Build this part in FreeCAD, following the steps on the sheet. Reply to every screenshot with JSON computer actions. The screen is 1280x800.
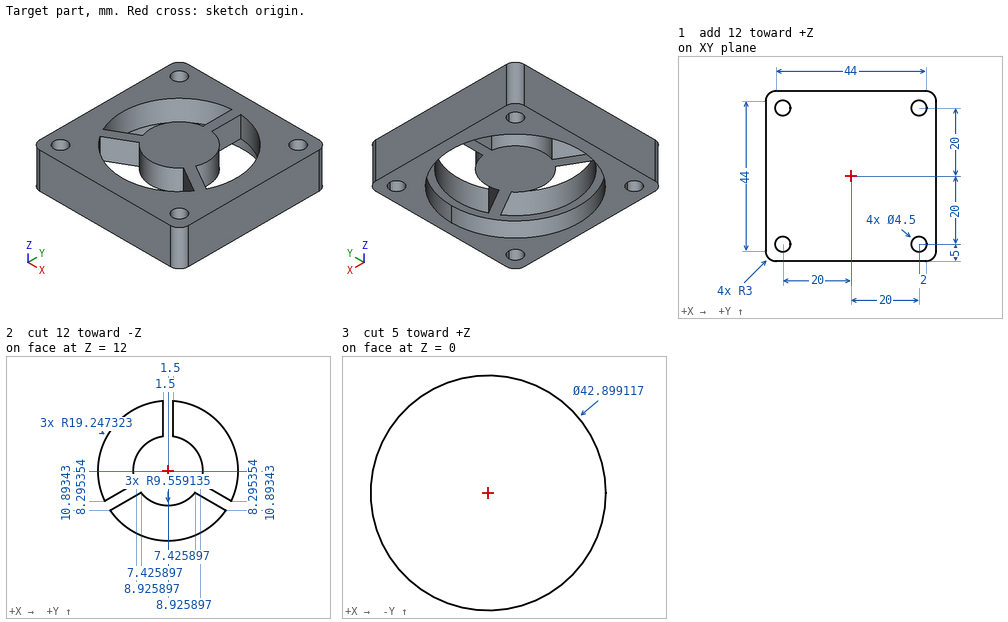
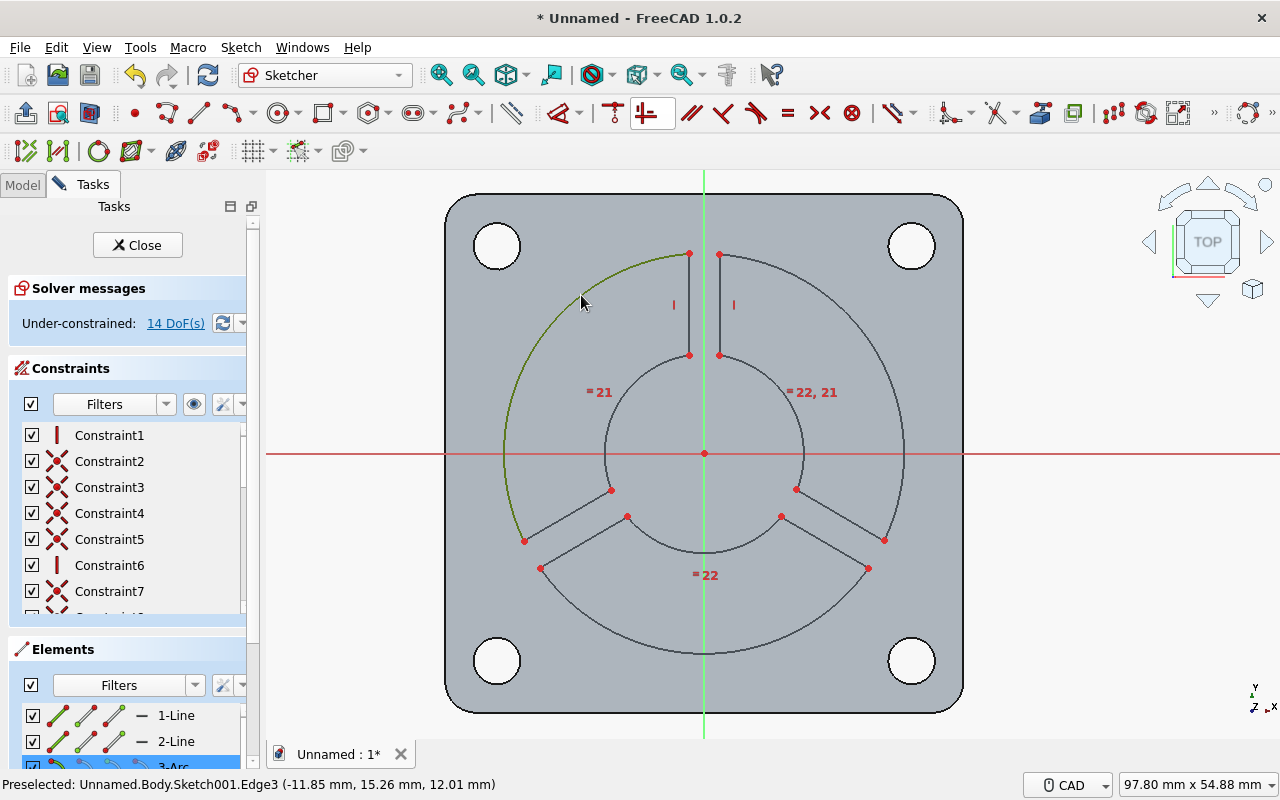
{"action": "left_click", "coordinate": [902, 428]}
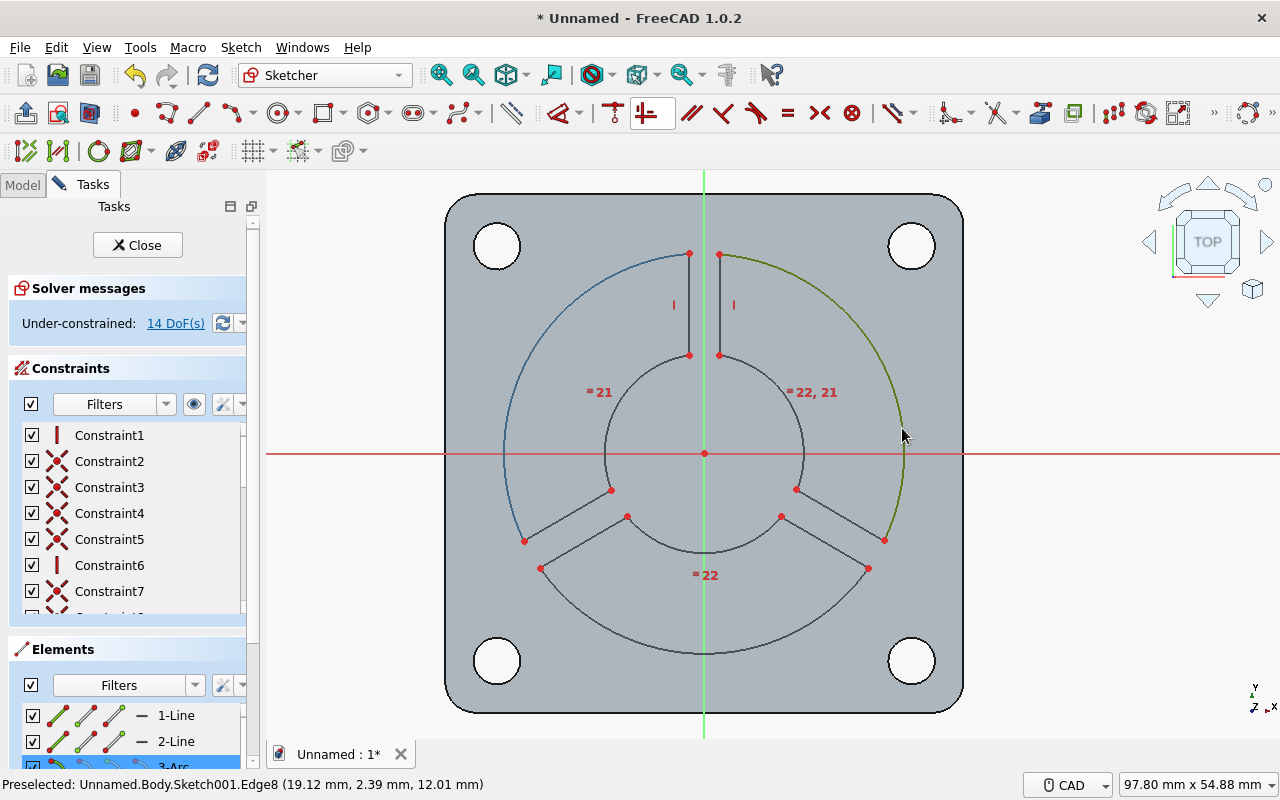
{"action": "left_click", "coordinate": [629, 639]}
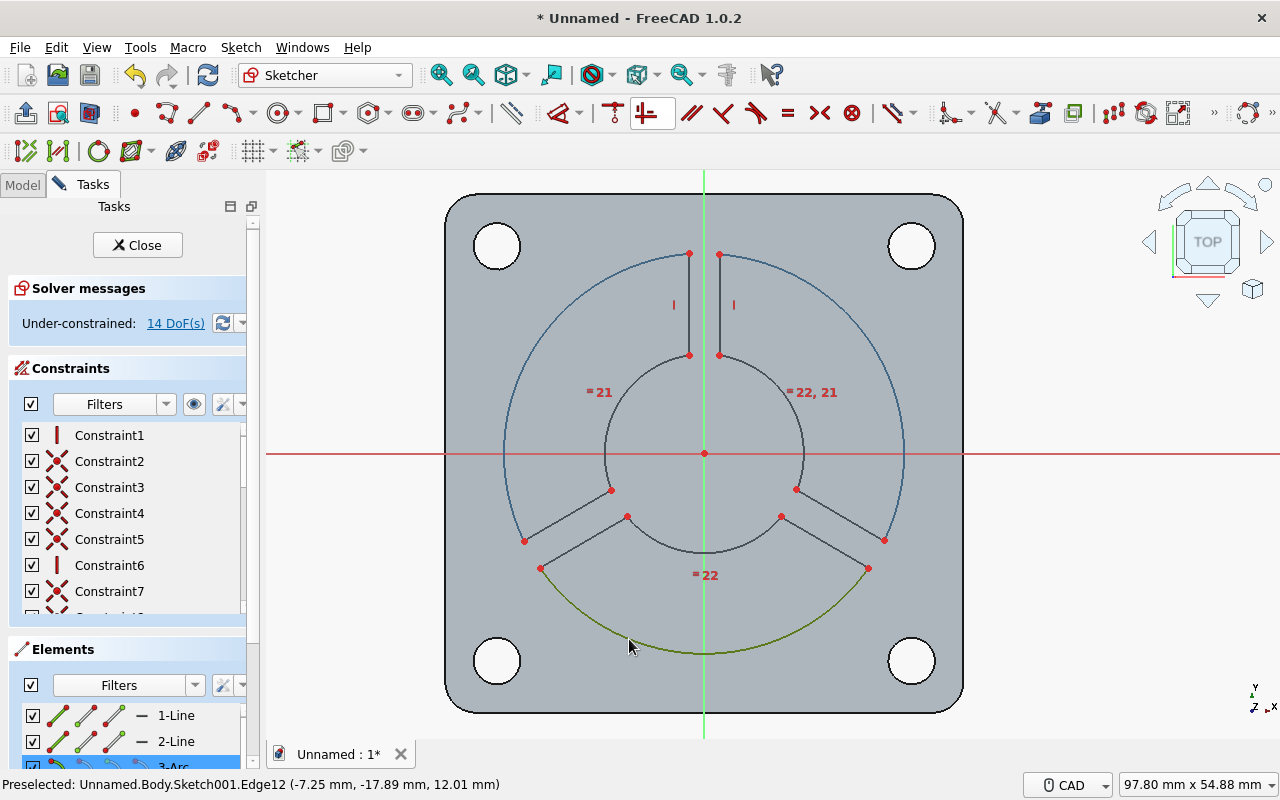
{"action": "left_click", "coordinate": [788, 114]}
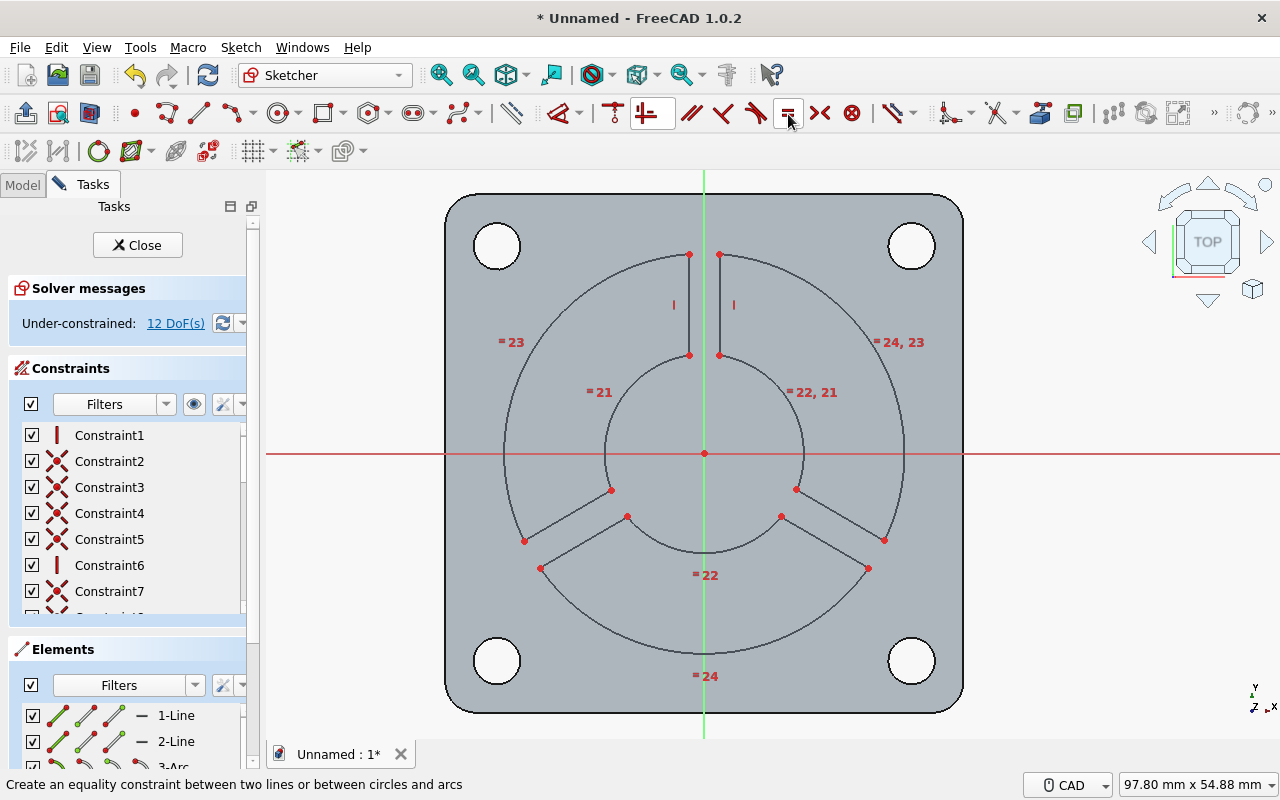
{"action": "left_click", "coordinate": [558, 114]}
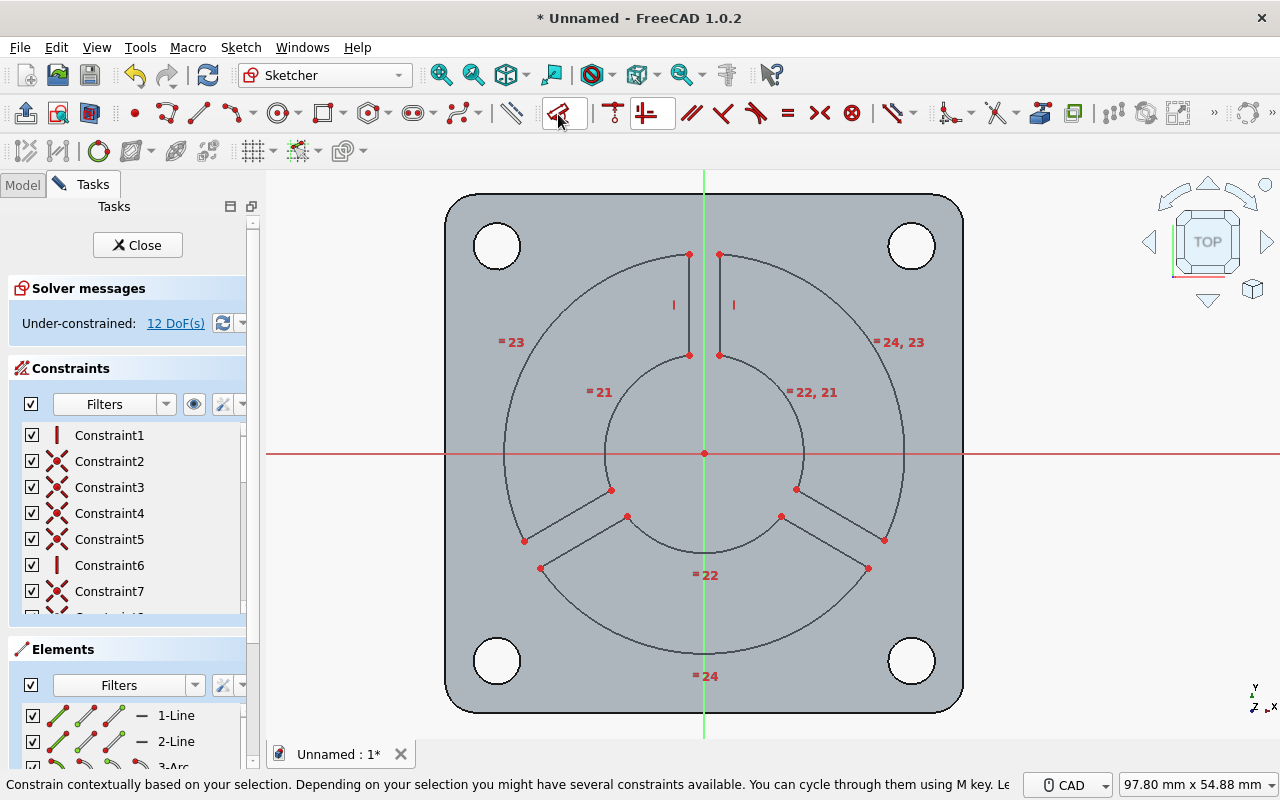
{"action": "left_click", "coordinate": [582, 296]}
{"action": "left_click", "coordinate": [562, 271]}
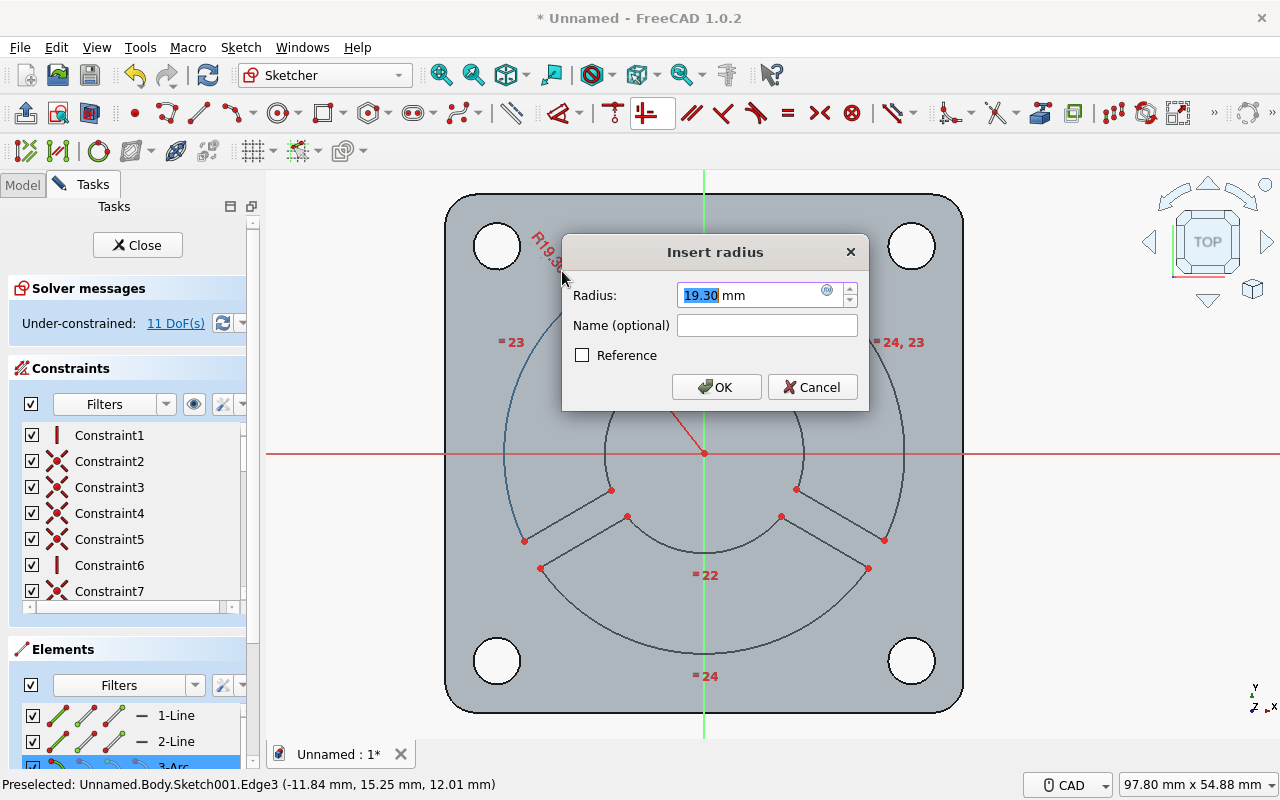
{"action": "type", "text": "19.247323"}
{"action": "key", "text": "Return"}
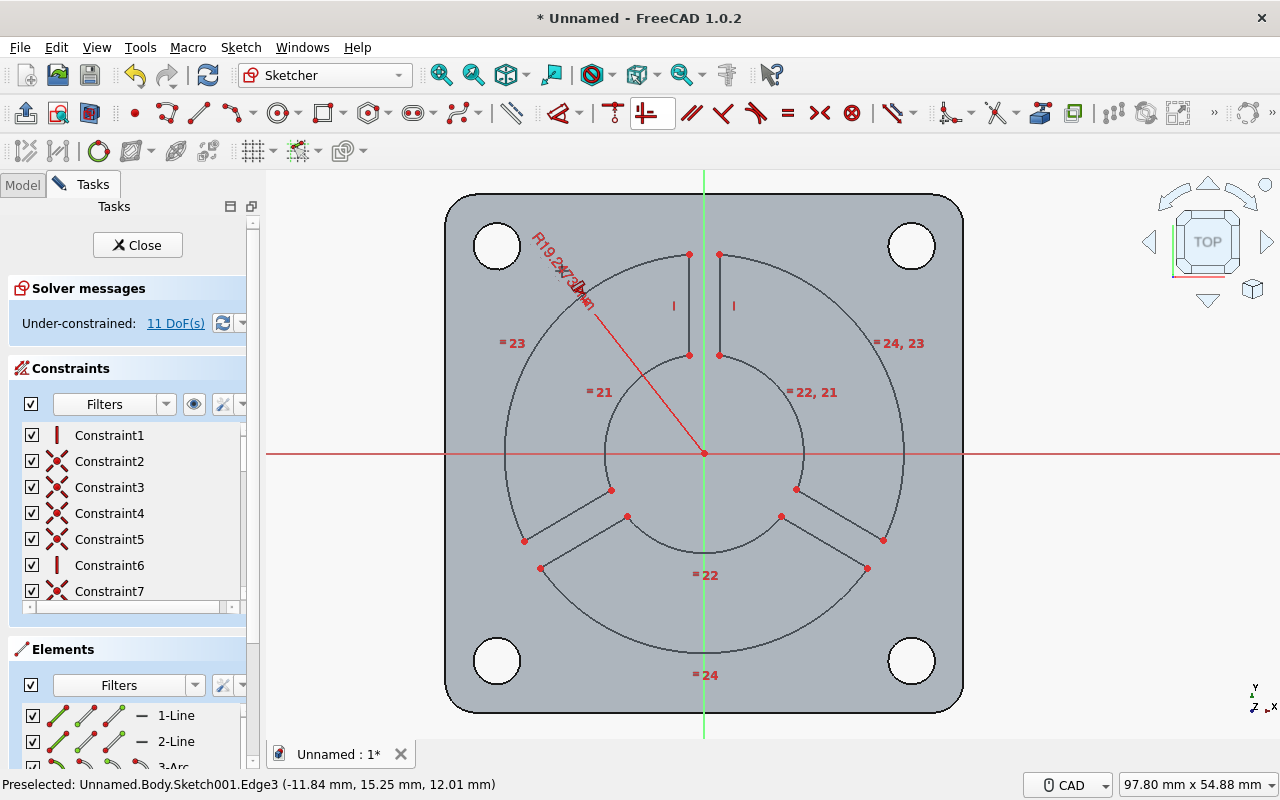
{"action": "left_click", "coordinate": [641, 377]}
{"action": "left_click", "coordinate": [621, 352]}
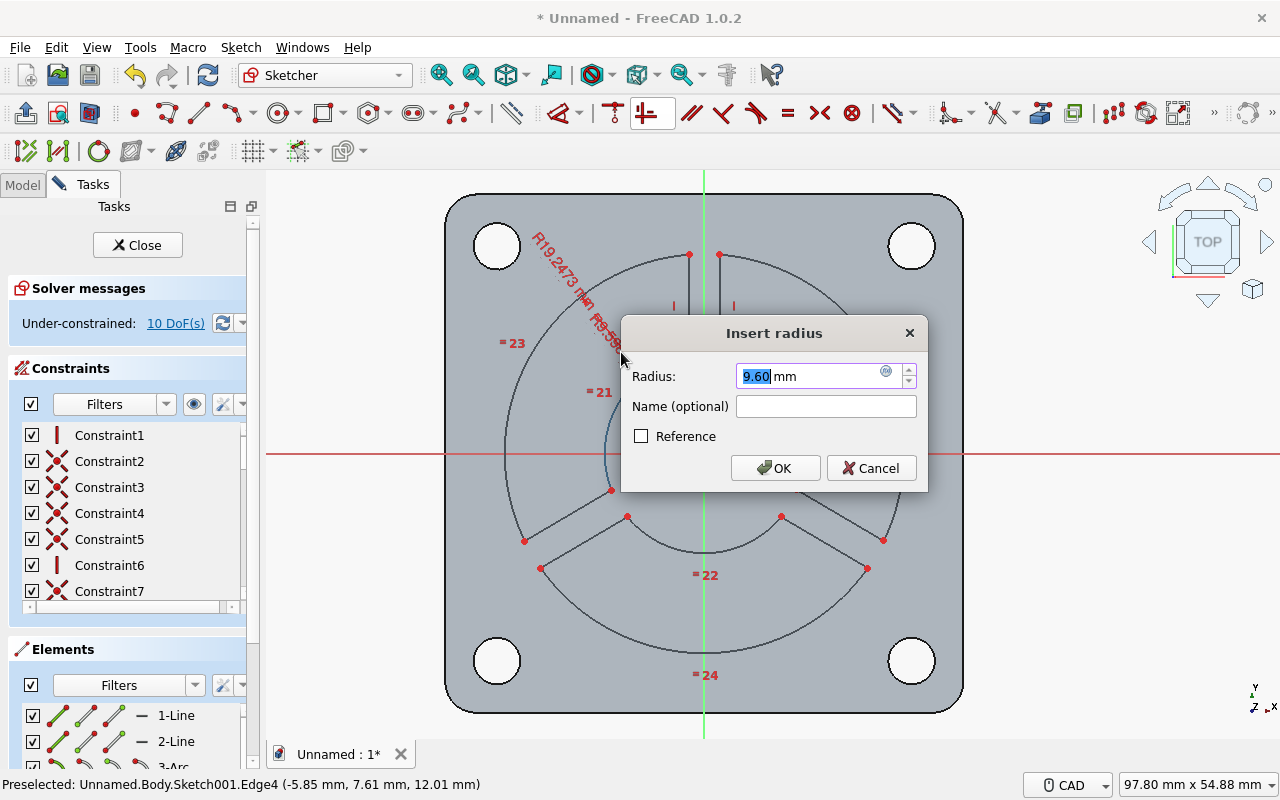
{"action": "type", "text": "9.559135"}
{"action": "key", "text": "Return"}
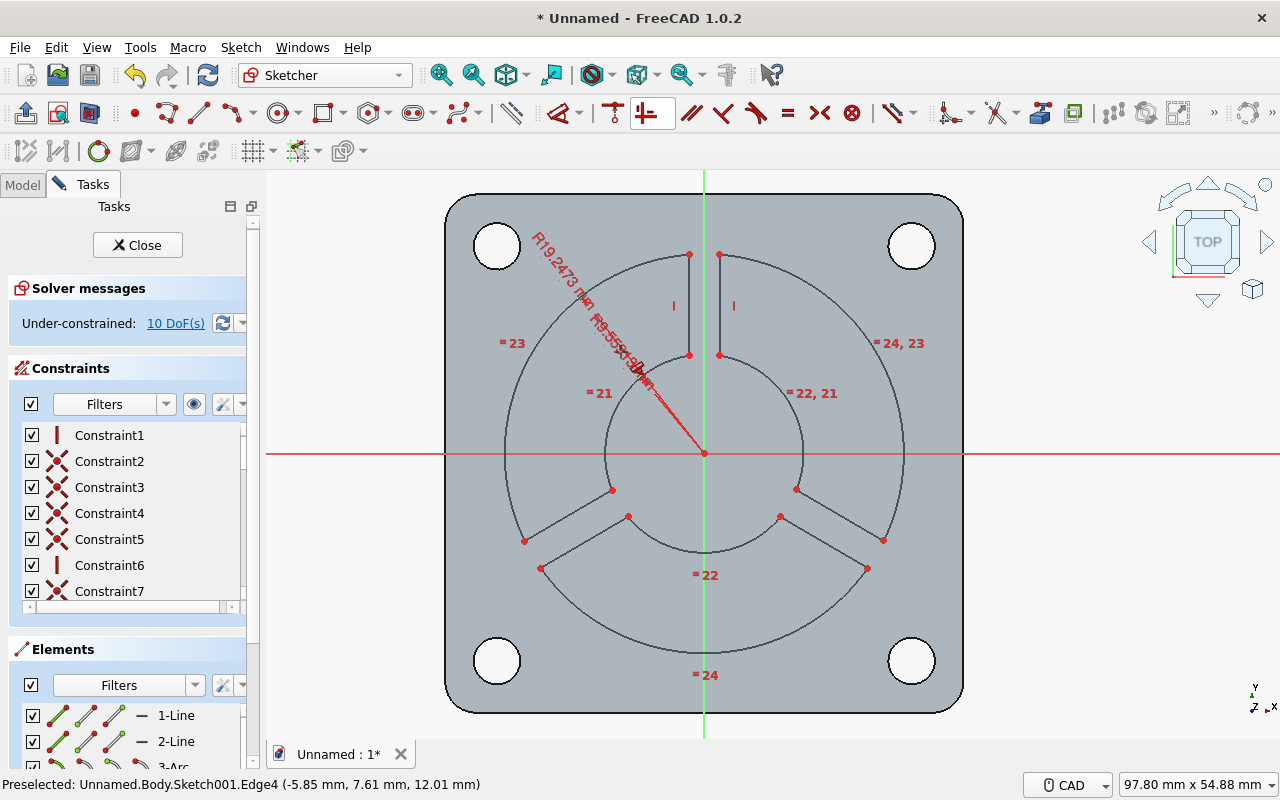
{"action": "scroll", "coordinate": [689, 356], "scroll_direction": "up", "scroll_amount": 5}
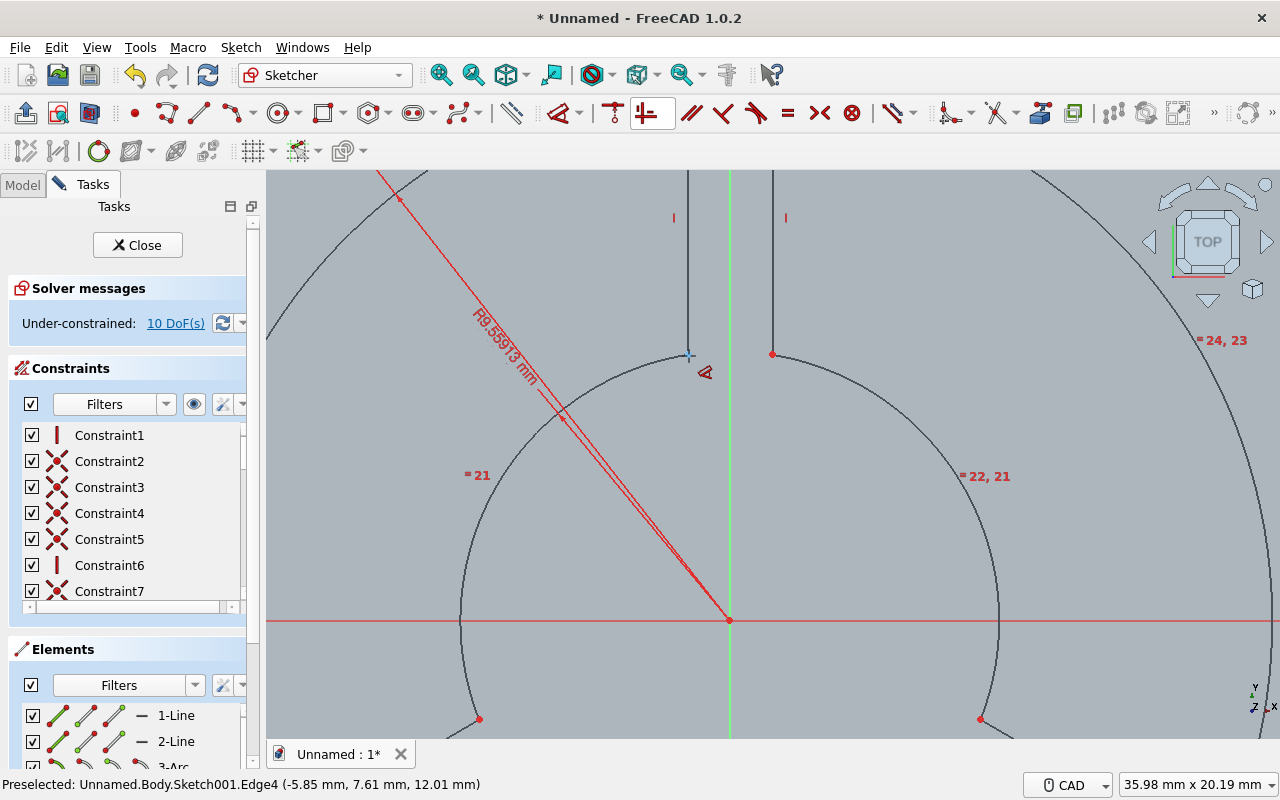
{"action": "left_click", "coordinate": [688, 355]}
{"action": "left_click", "coordinate": [709, 321]}